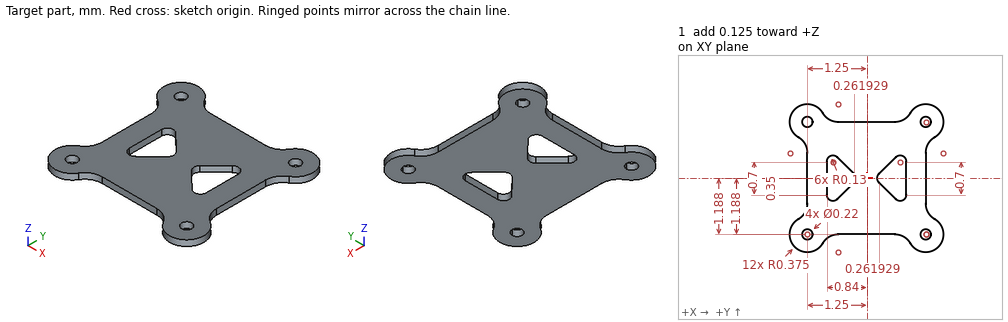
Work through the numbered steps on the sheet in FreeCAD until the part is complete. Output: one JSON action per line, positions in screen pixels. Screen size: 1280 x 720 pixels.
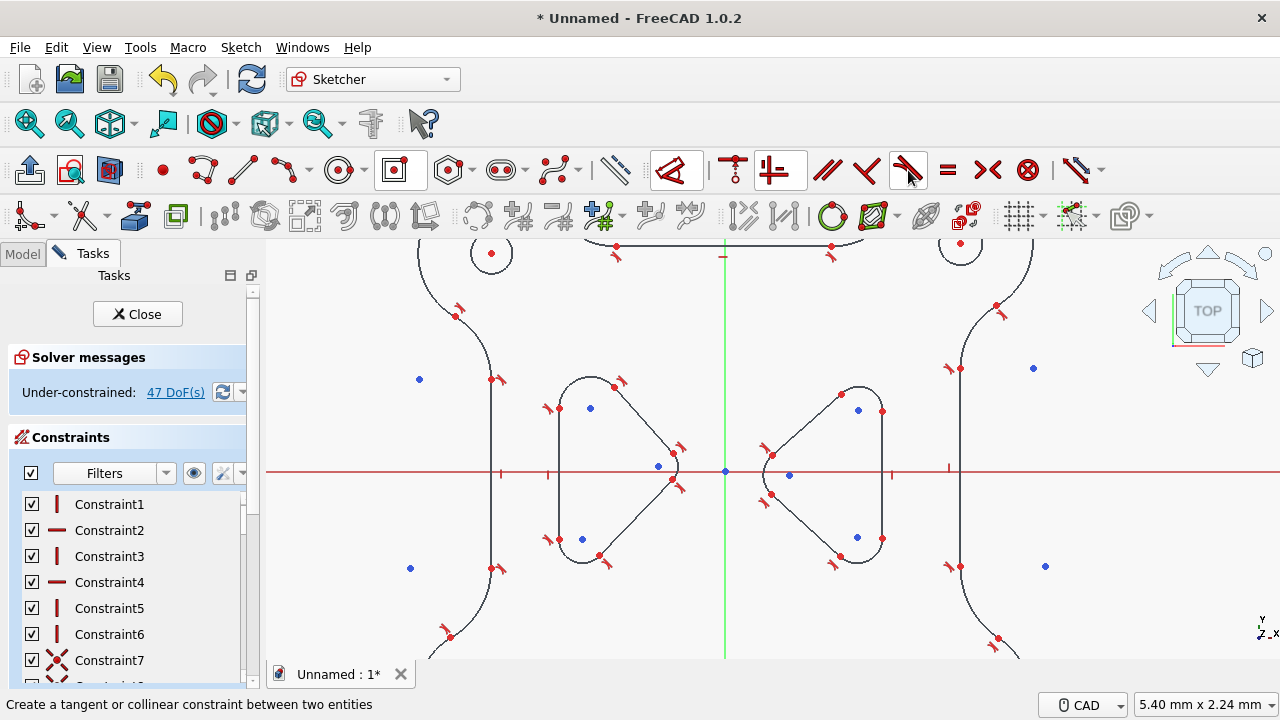
{"action": "left_click", "coordinate": [793, 437]}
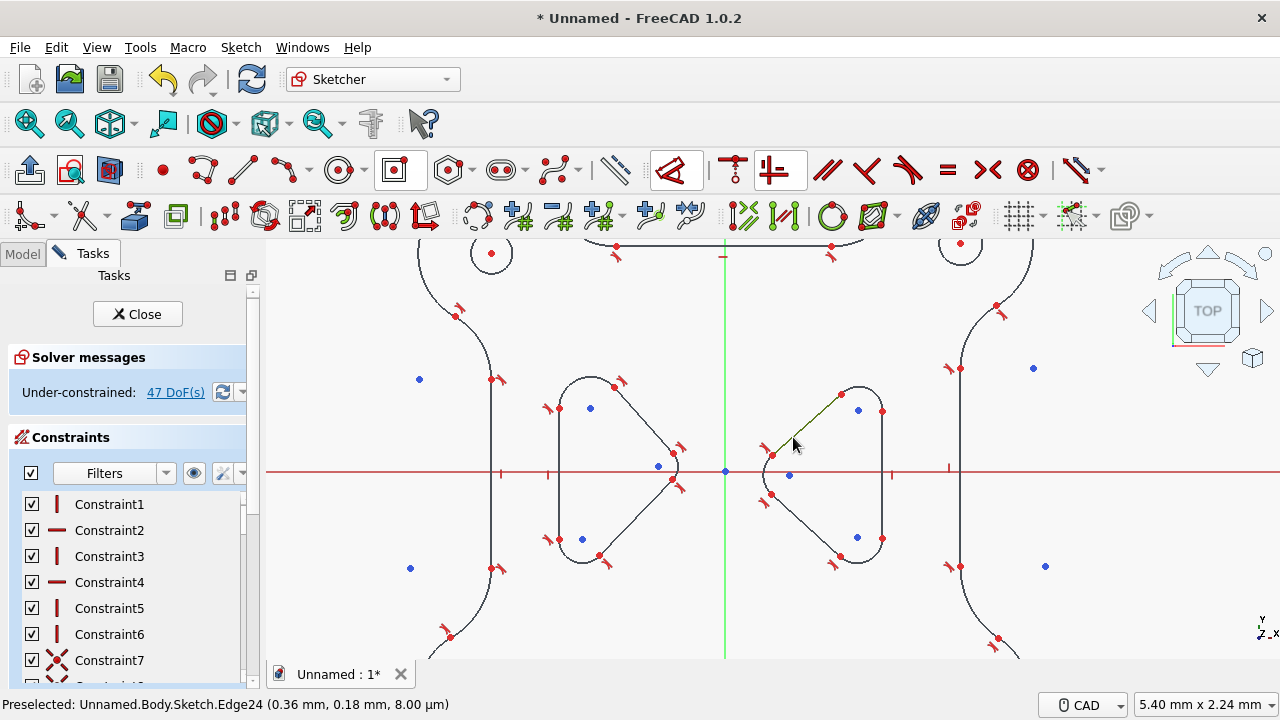
{"action": "left_click", "coordinate": [877, 395]}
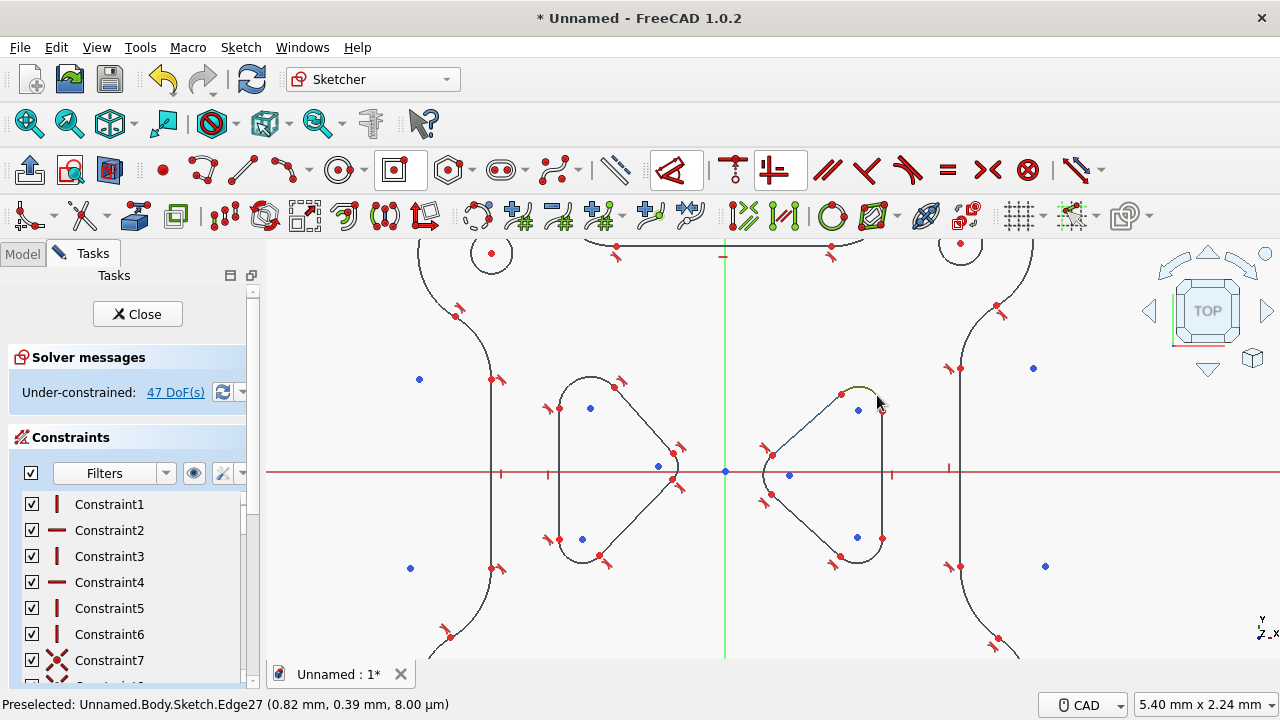
{"action": "left_click", "coordinate": [908, 170]}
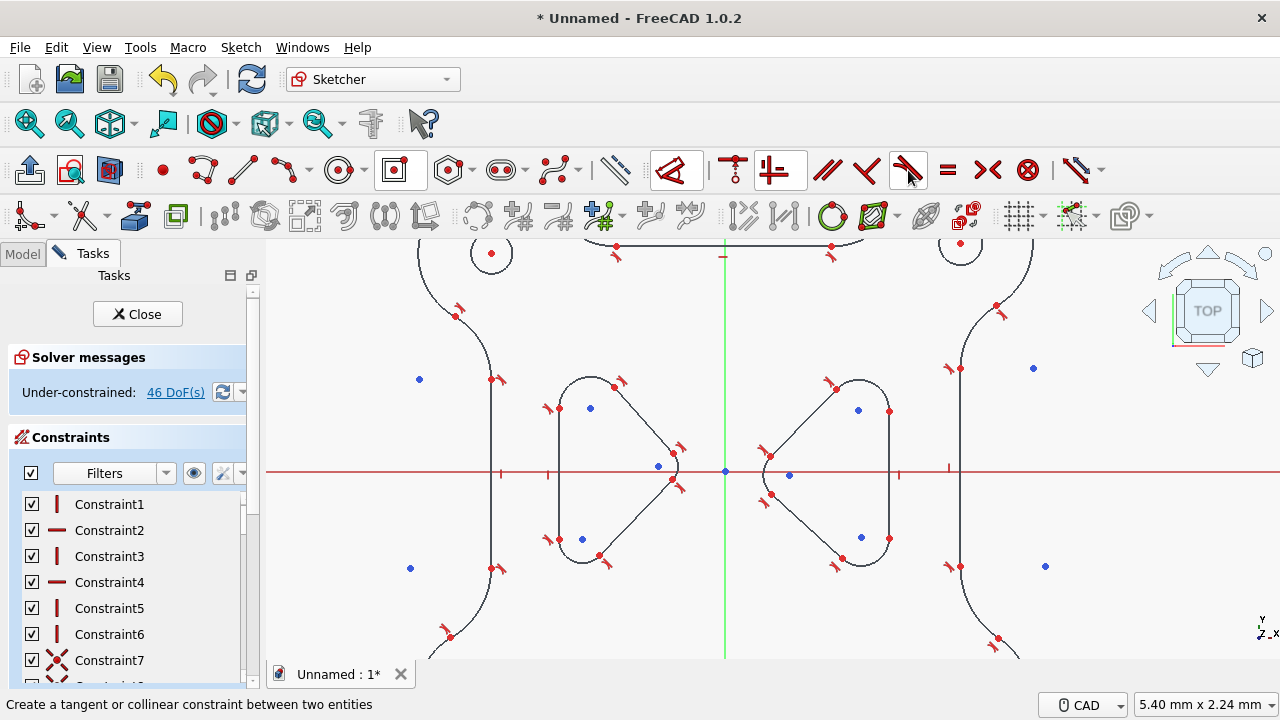
{"action": "left_click", "coordinate": [889, 449]}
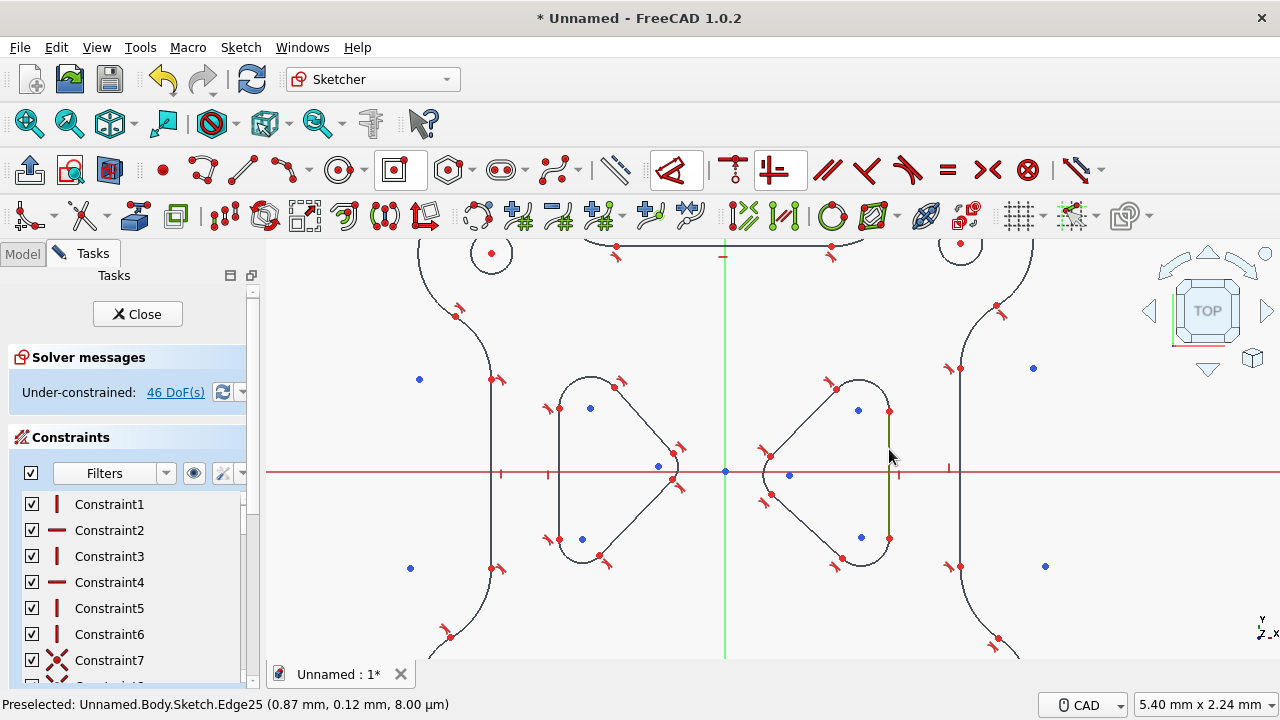
{"action": "left_click", "coordinate": [882, 391]}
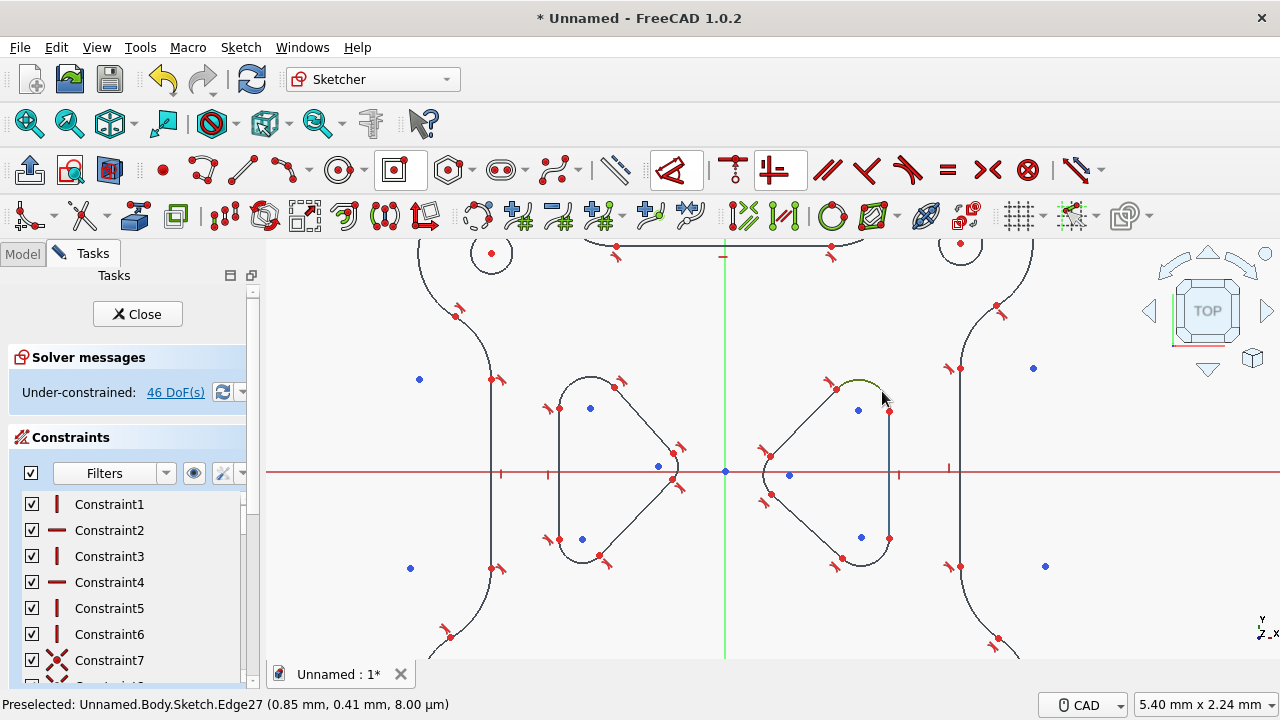
{"action": "left_click", "coordinate": [908, 170]}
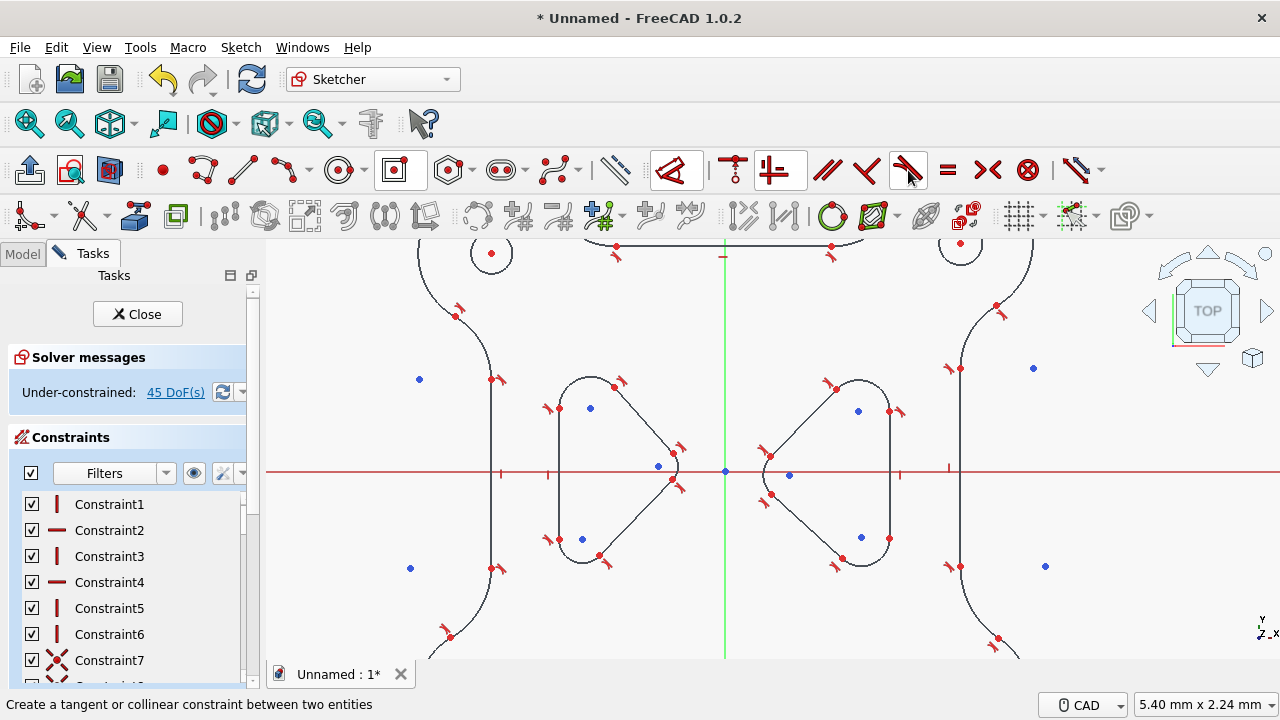
{"action": "left_click", "coordinate": [890, 449]}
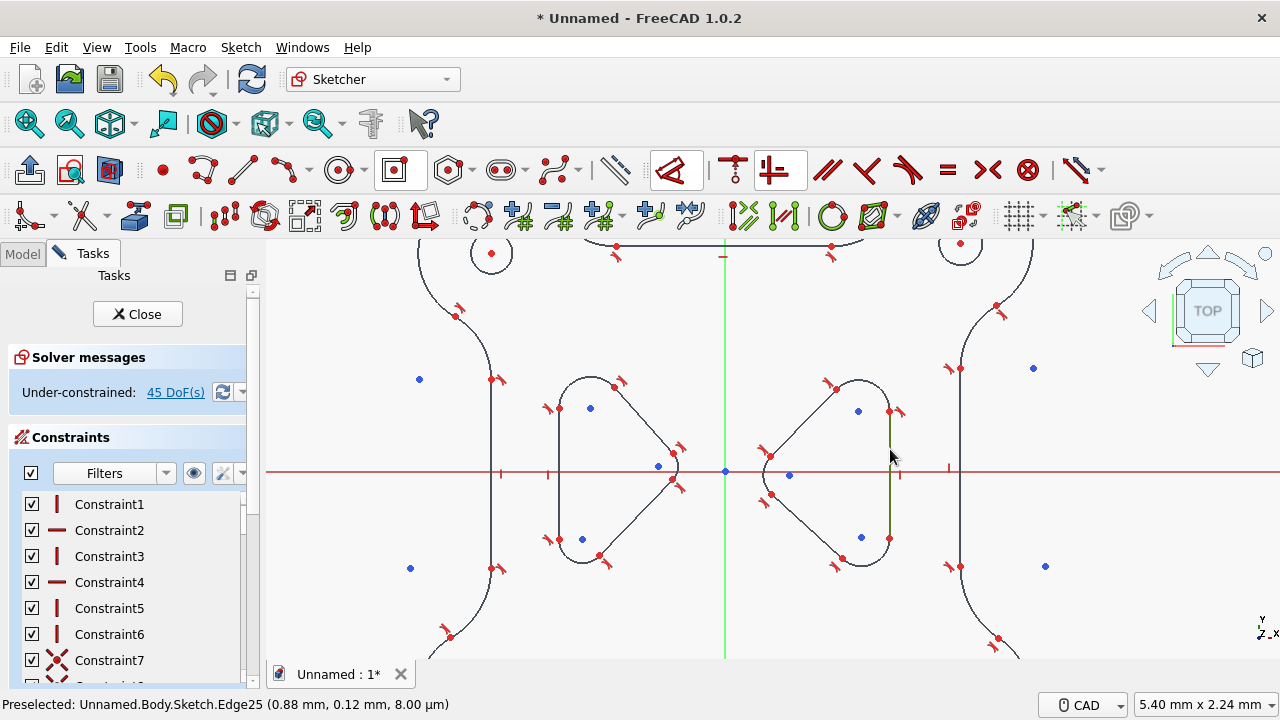
{"action": "left_click", "coordinate": [860, 566]}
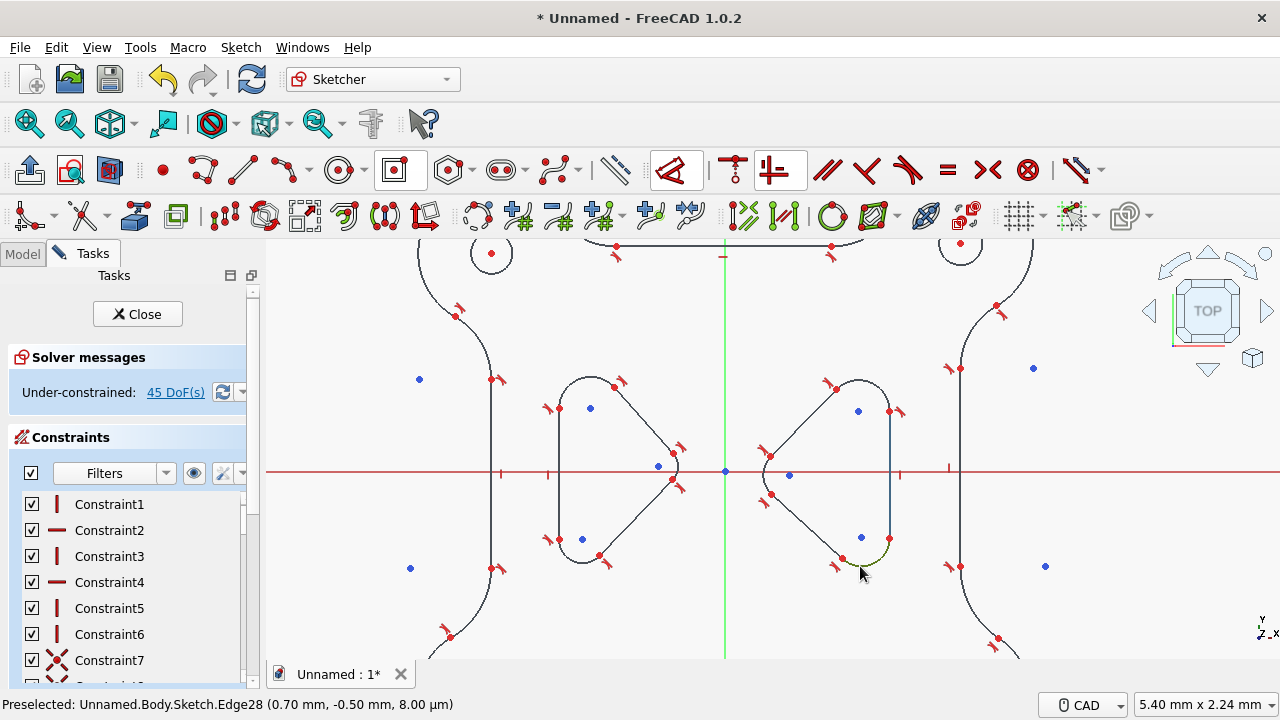
{"action": "left_click", "coordinate": [908, 170]}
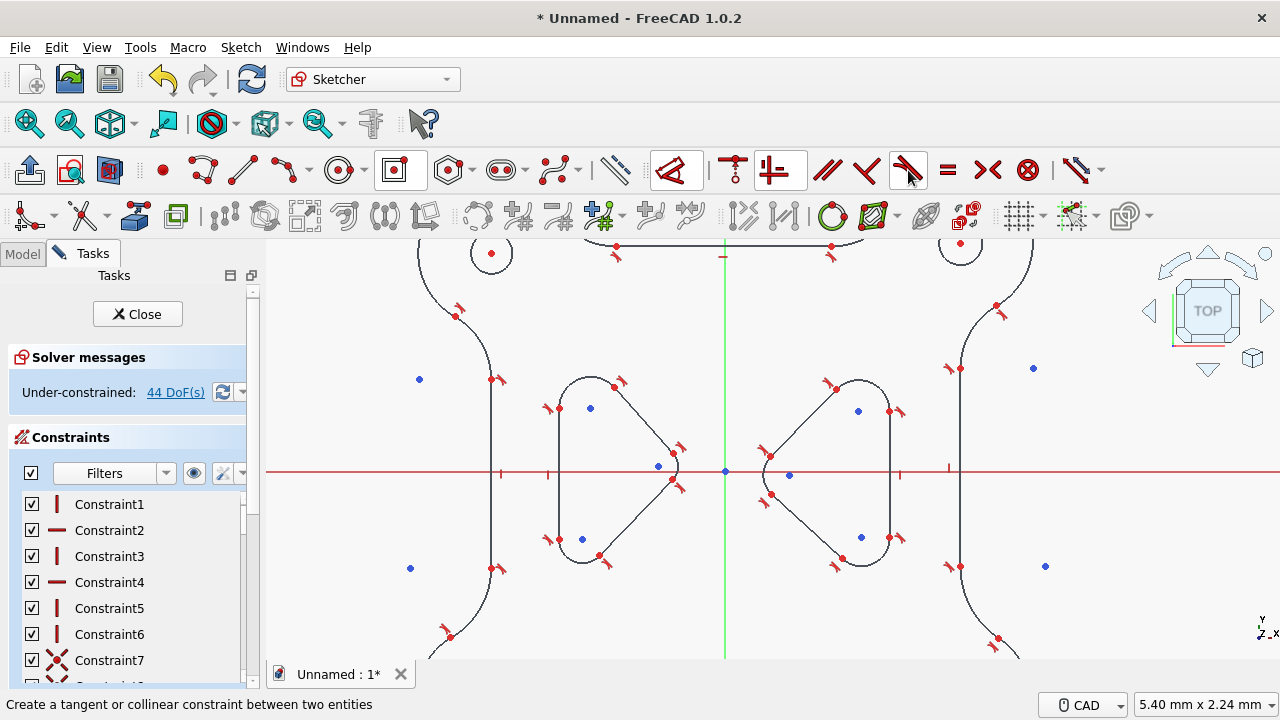
{"action": "left_click", "coordinate": [470, 622]}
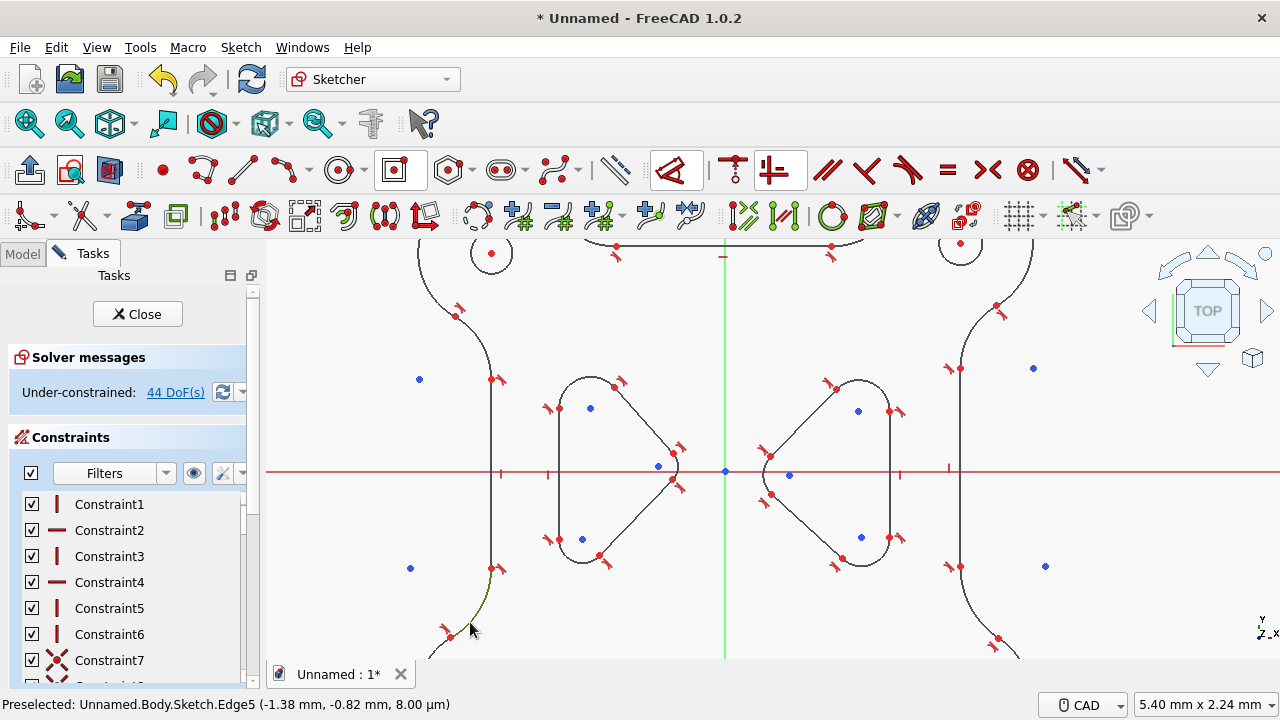
{"action": "scroll", "coordinate": [688, 430], "scroll_direction": "down", "scroll_amount": 4}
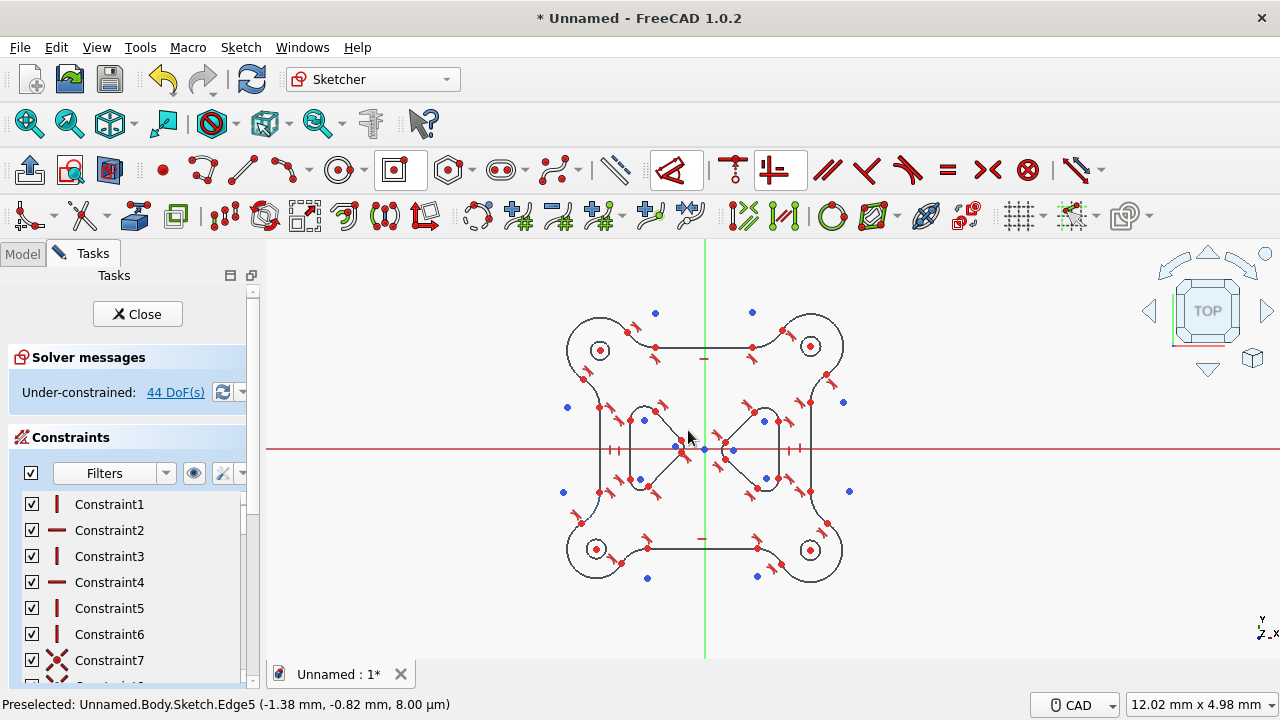
{"action": "left_click", "coordinate": [567, 551]}